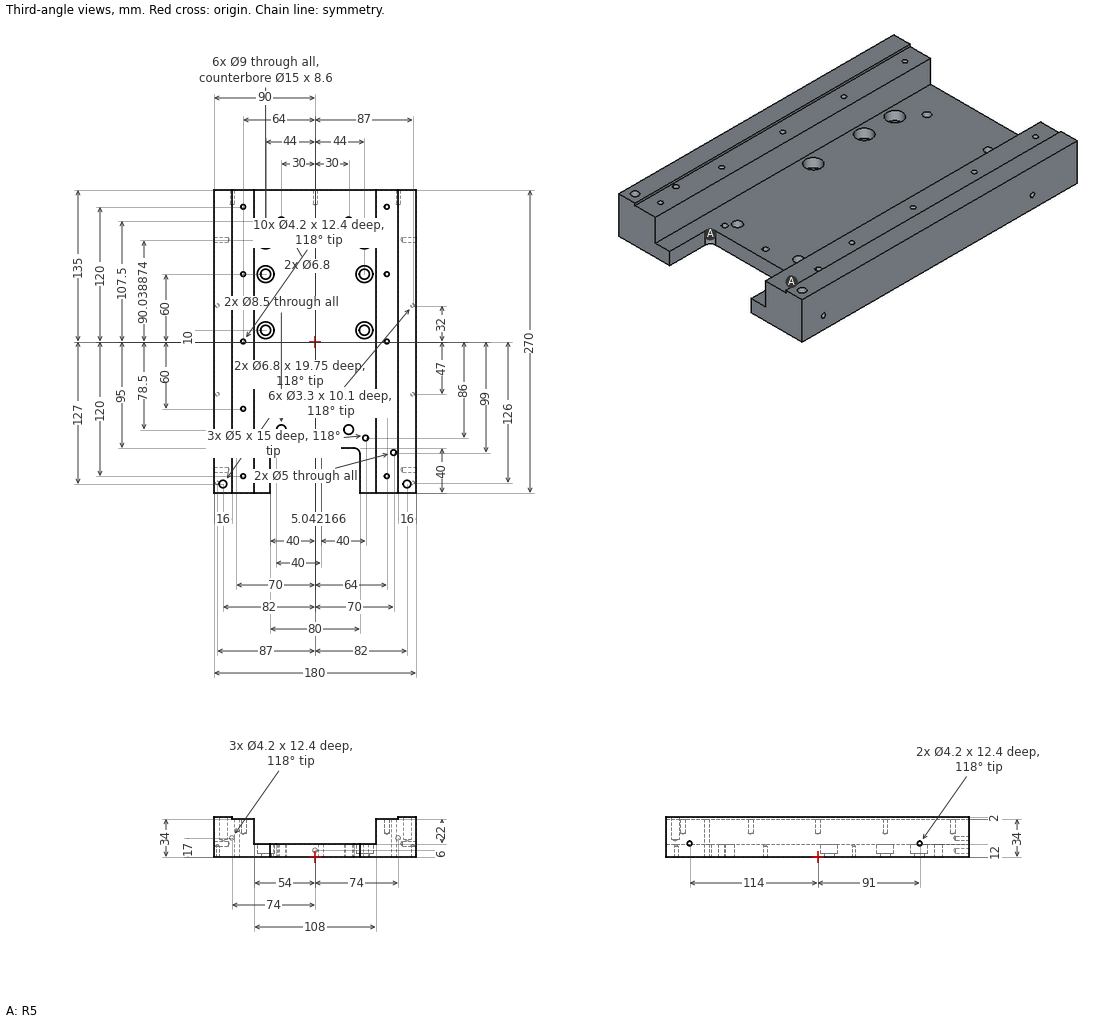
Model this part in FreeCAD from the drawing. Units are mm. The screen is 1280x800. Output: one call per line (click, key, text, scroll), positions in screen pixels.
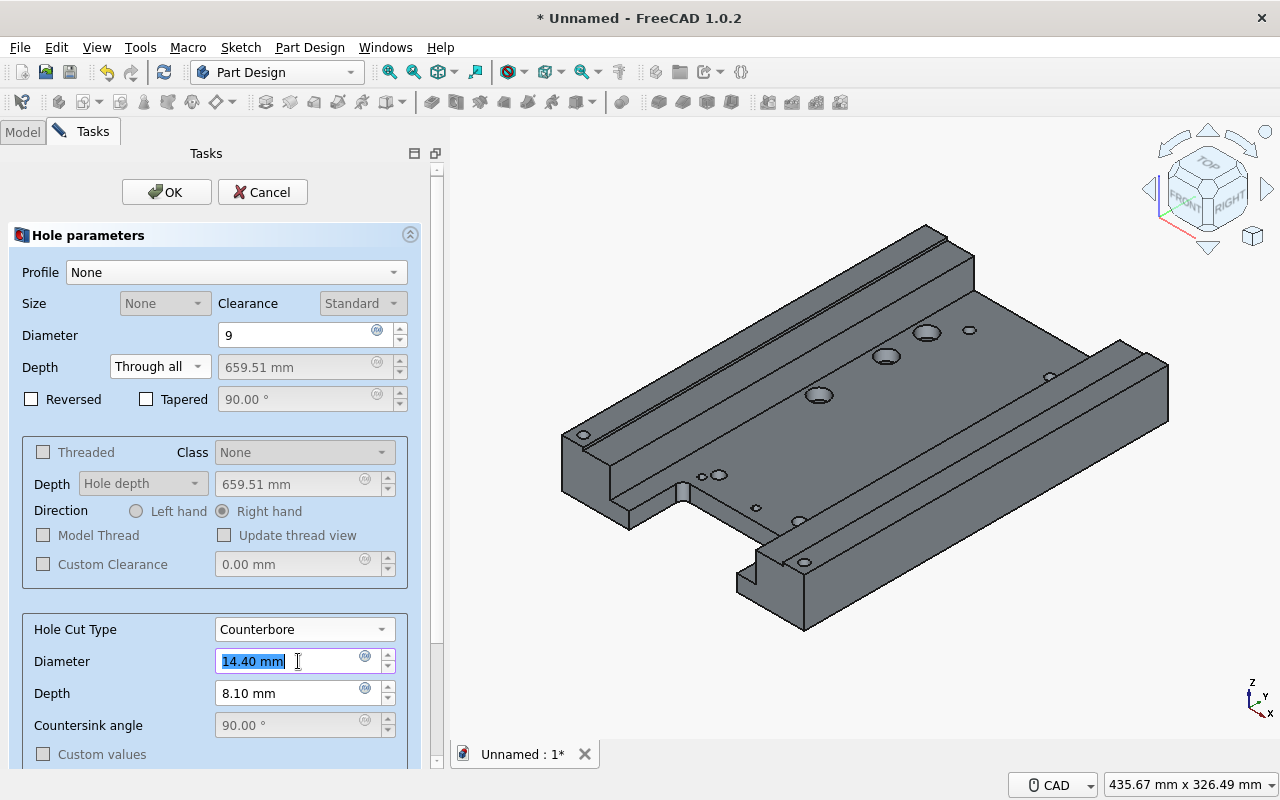
text(15)
key(Tab)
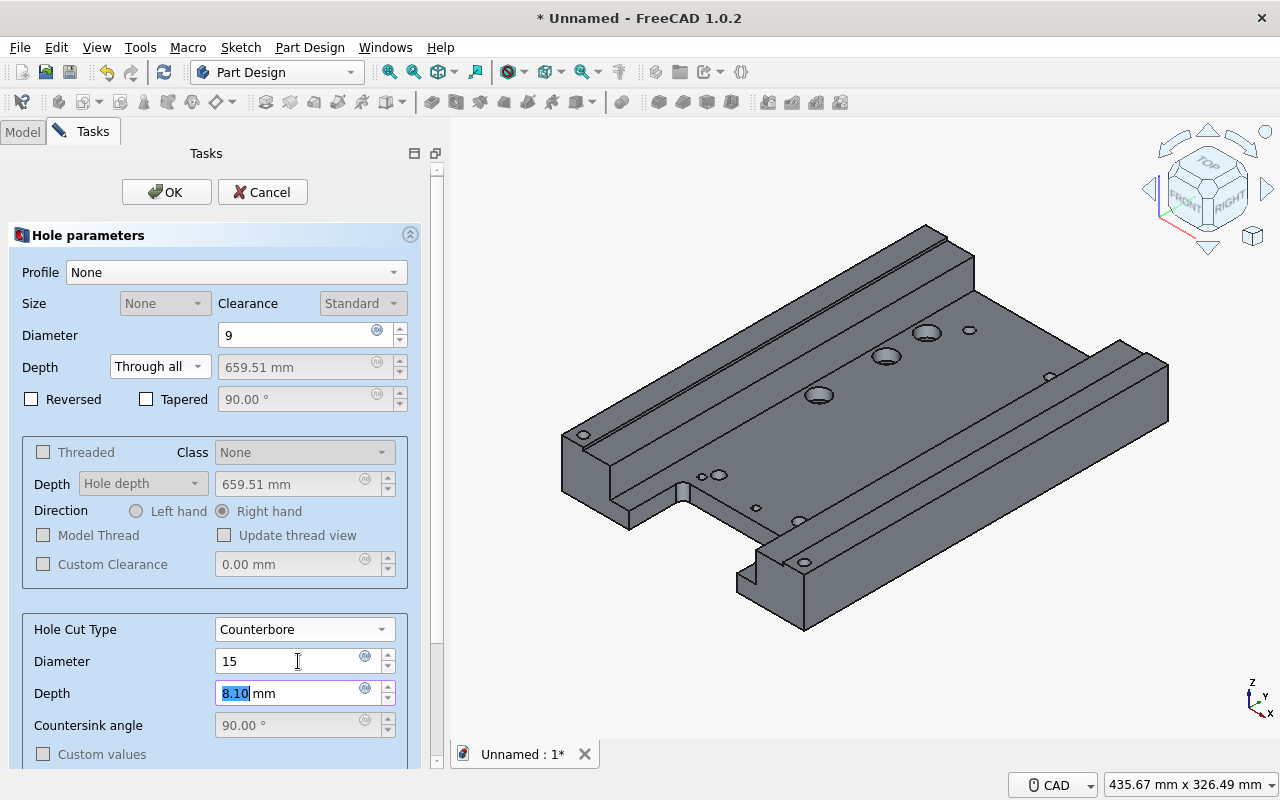
text(8.6)
key(Tab)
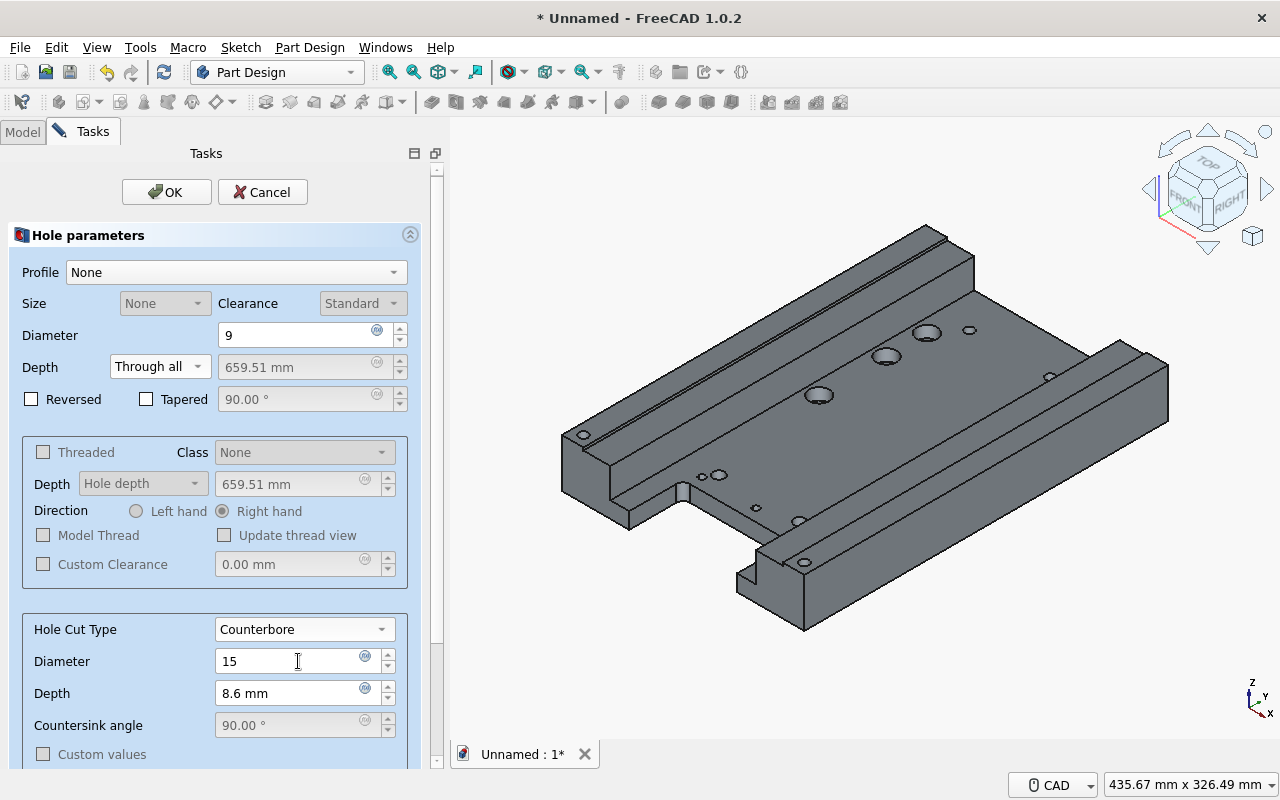
click(167, 192)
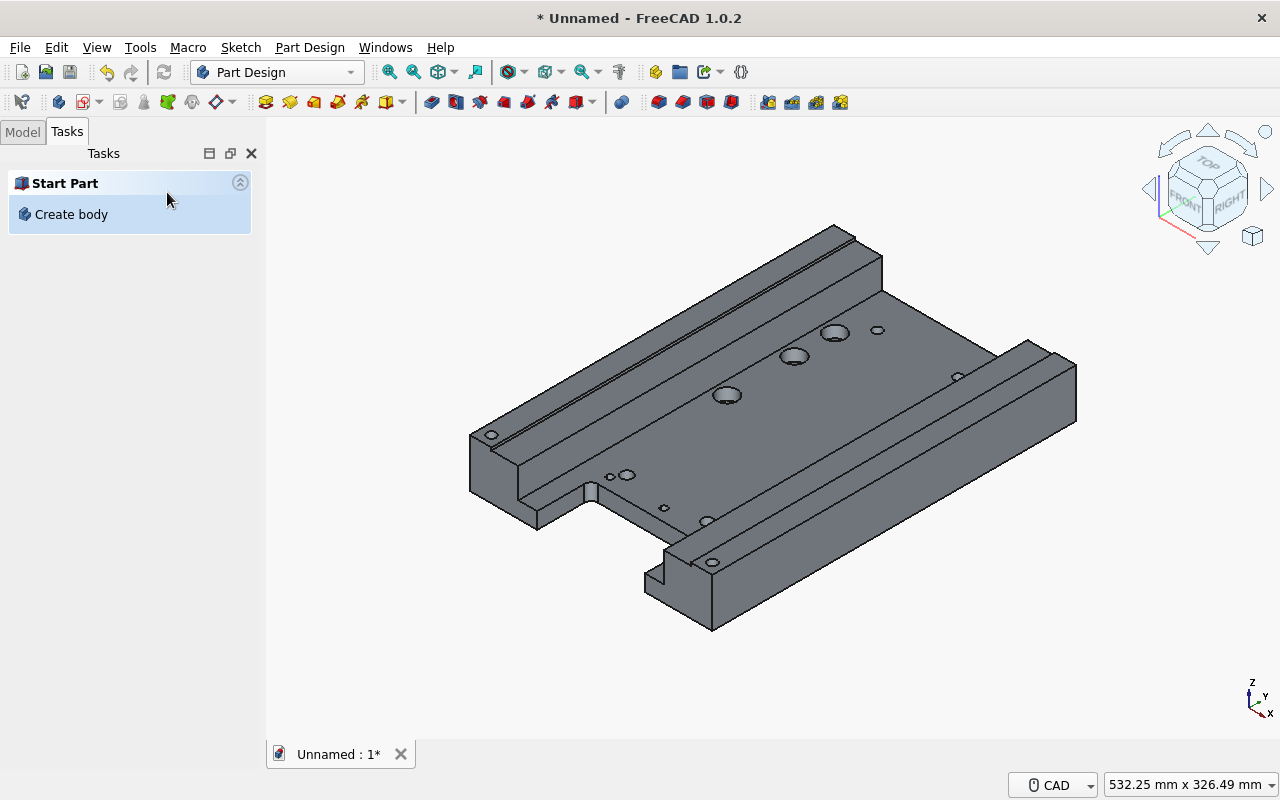
key(6)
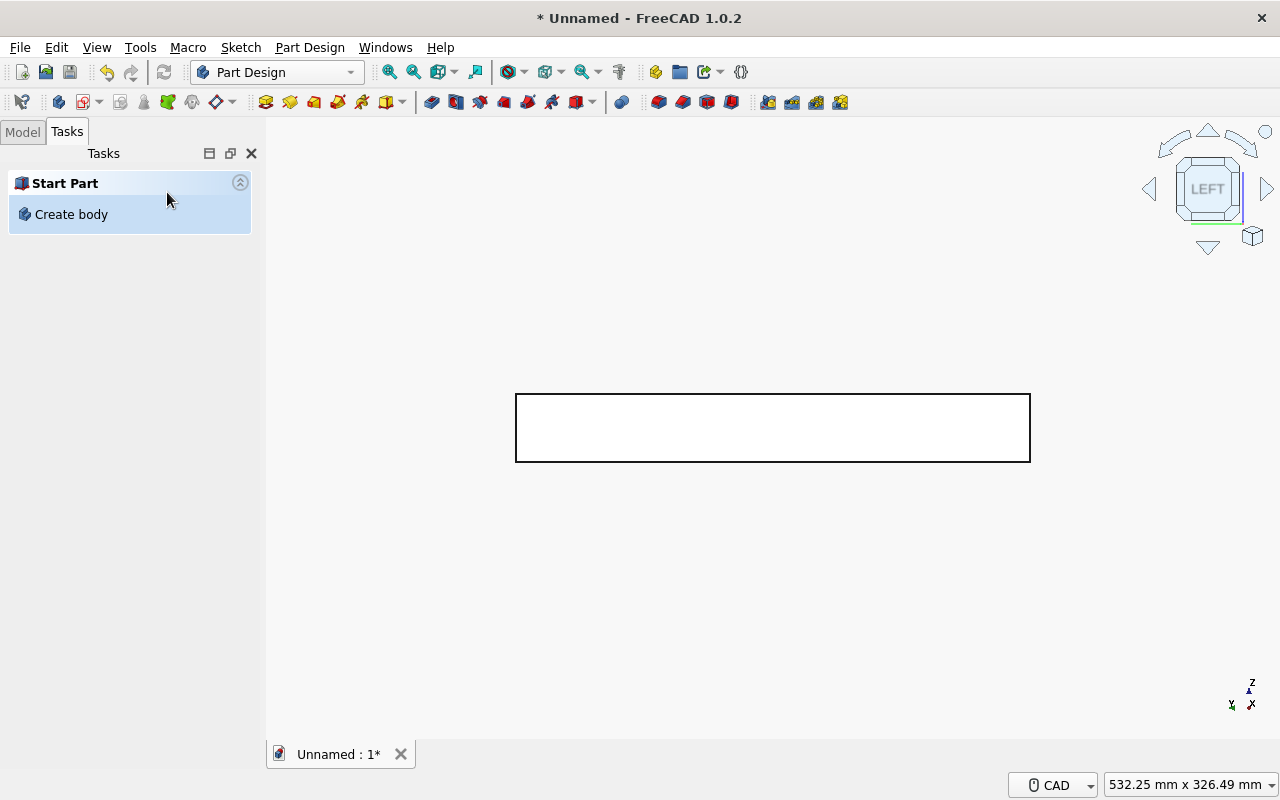
click(553, 427)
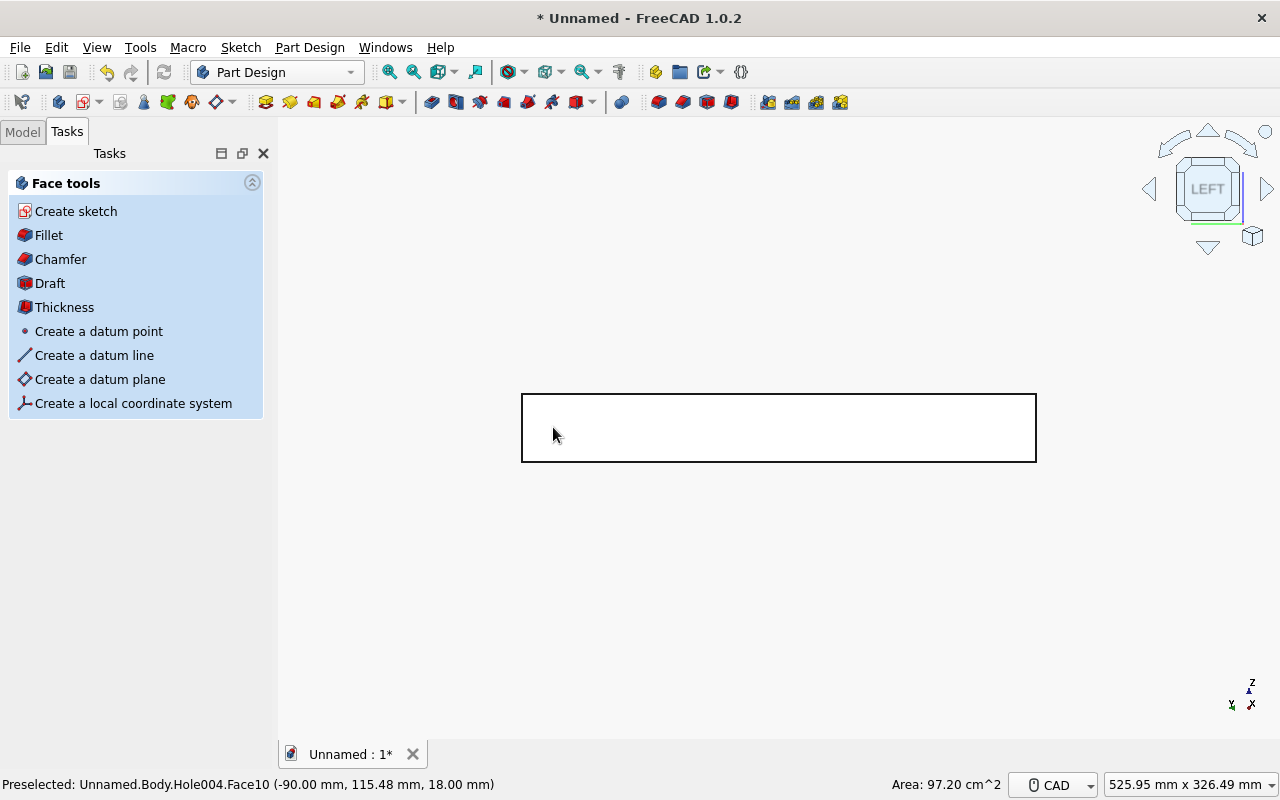
click(84, 102)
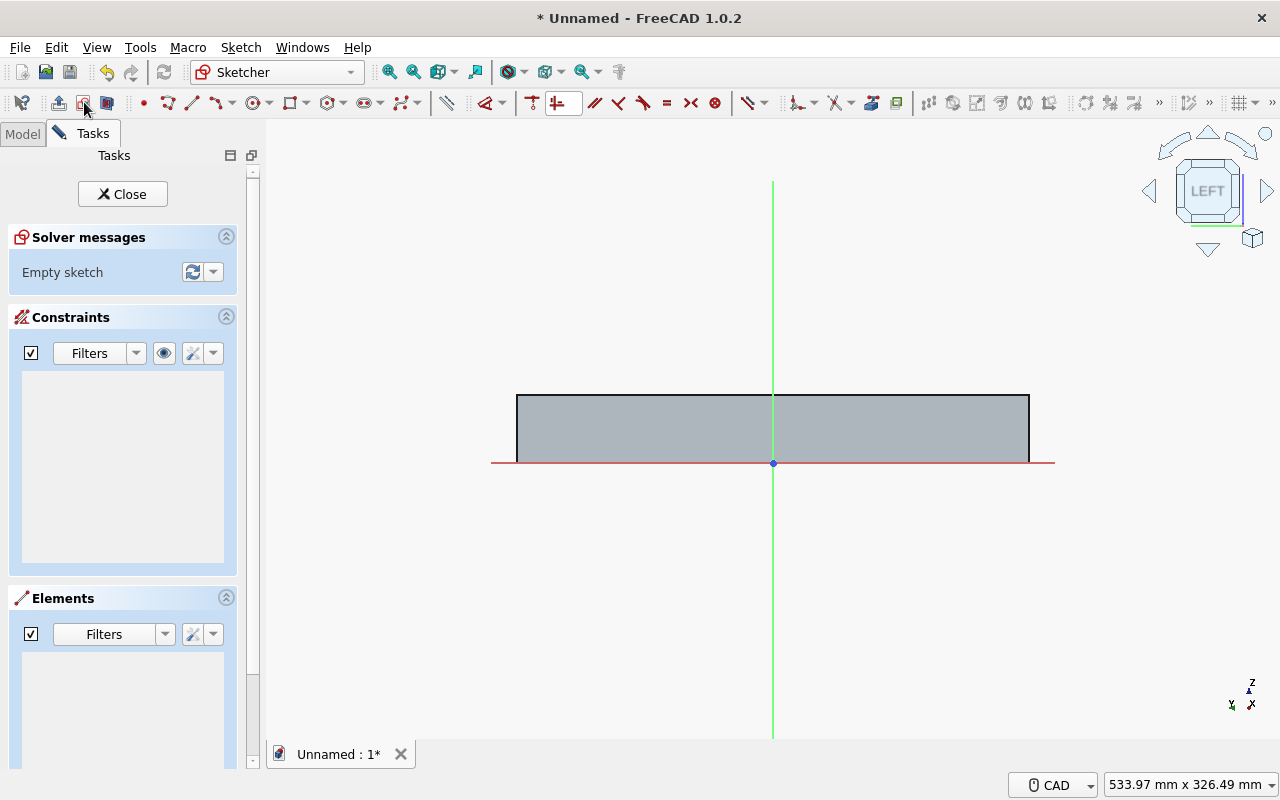
scroll(979, 492, up, 2)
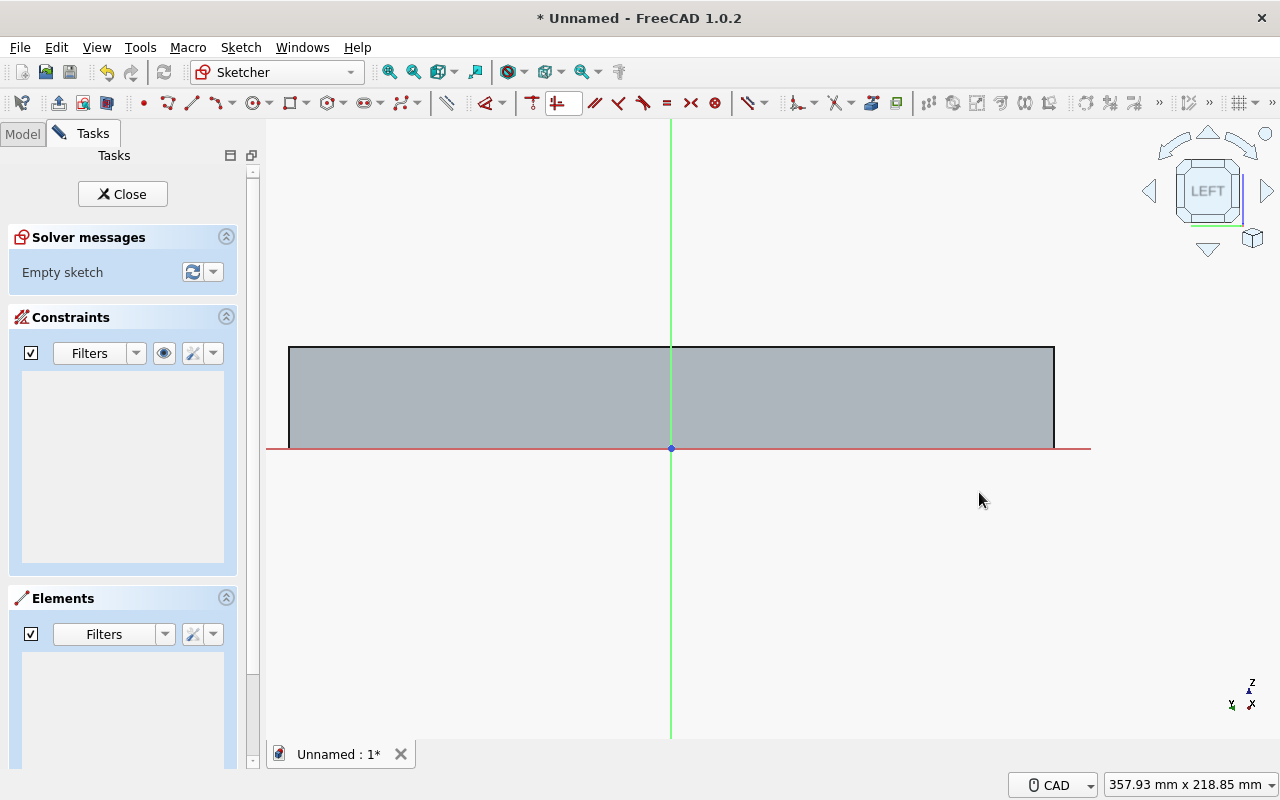
click(254, 104)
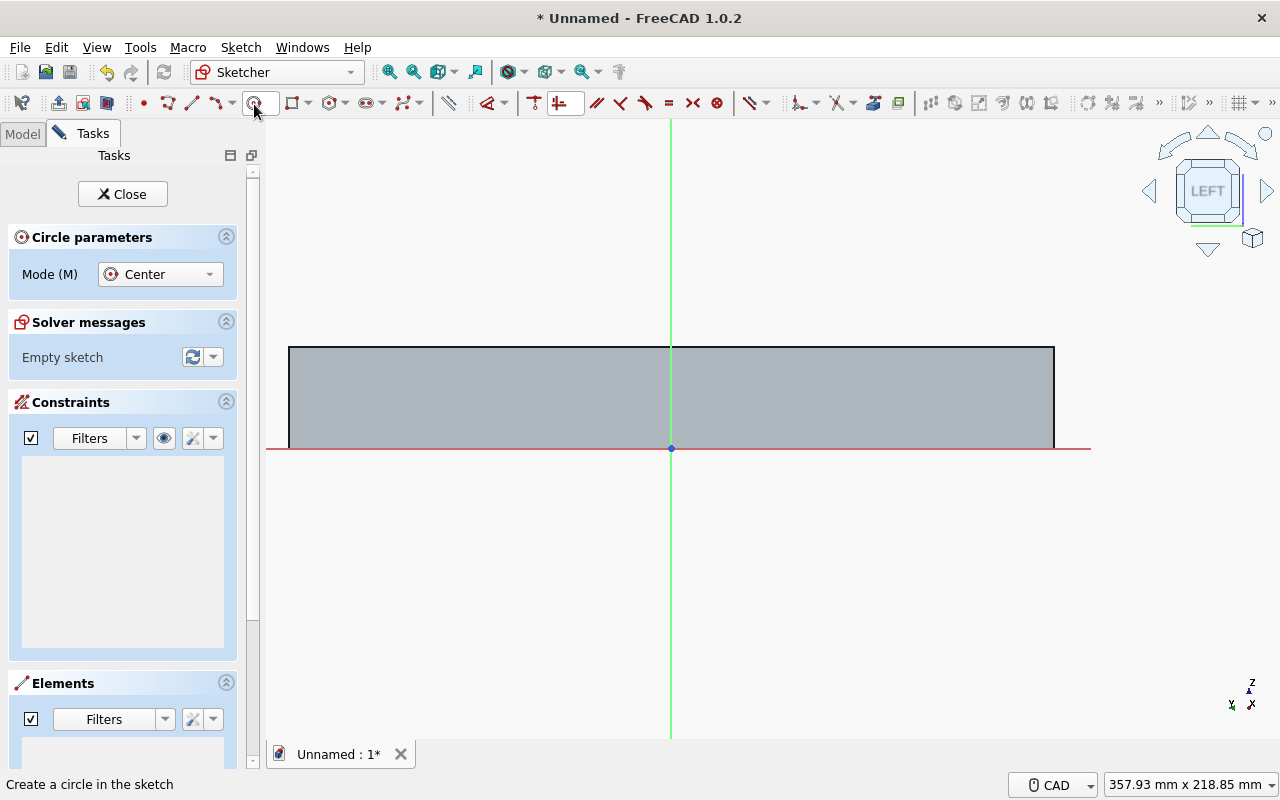
scroll(414, 415, up, 7)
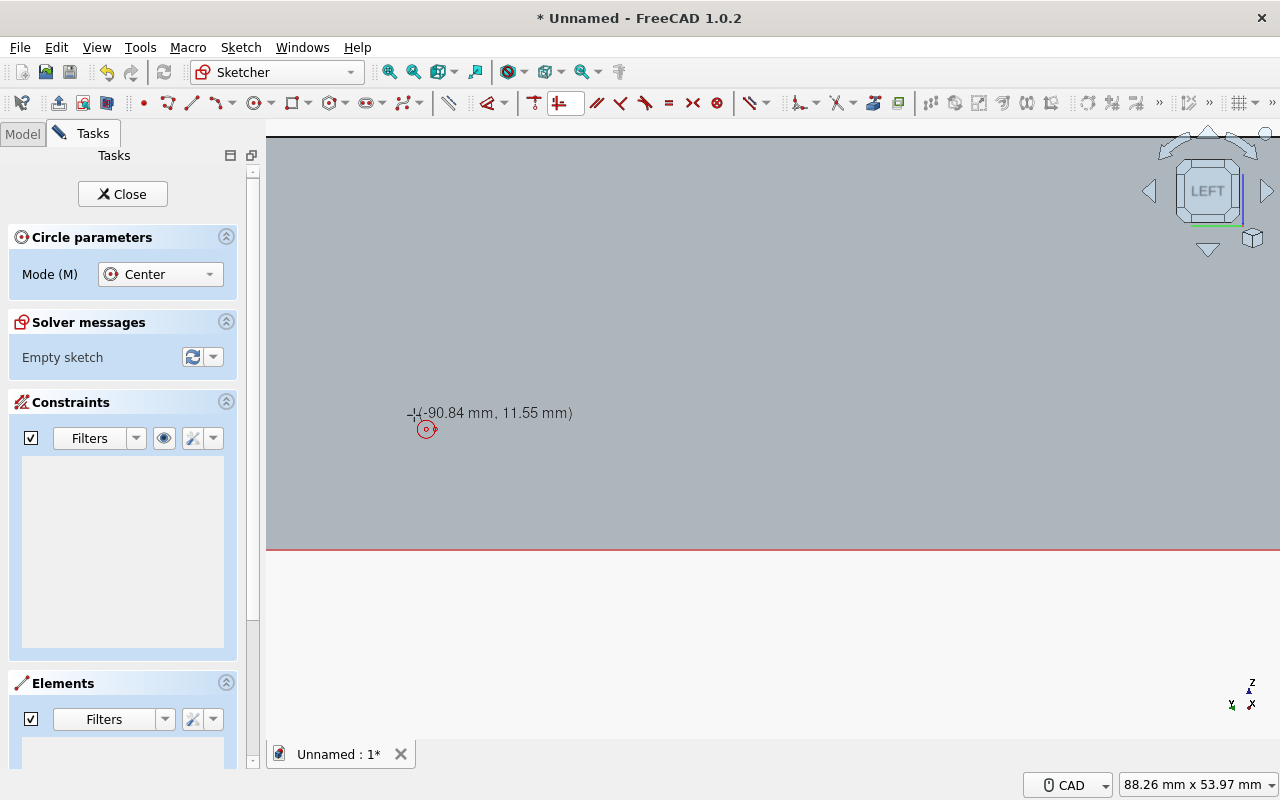
scroll(415, 416, down, 7)